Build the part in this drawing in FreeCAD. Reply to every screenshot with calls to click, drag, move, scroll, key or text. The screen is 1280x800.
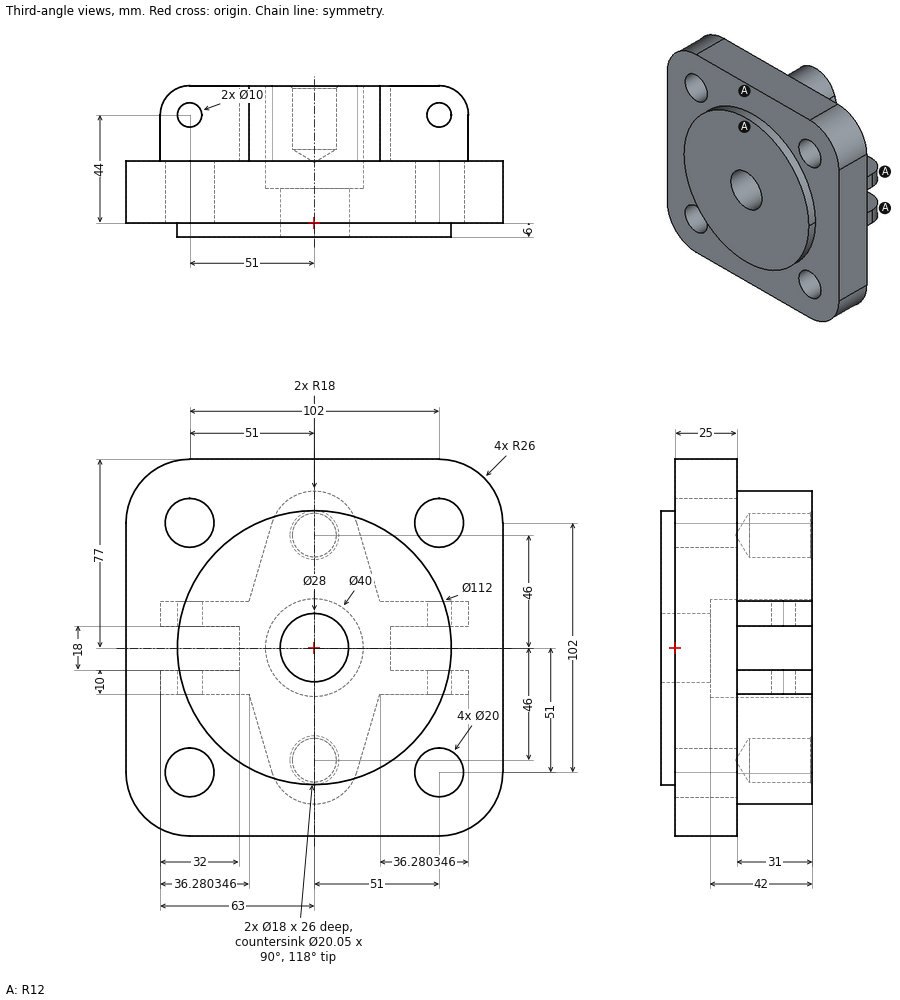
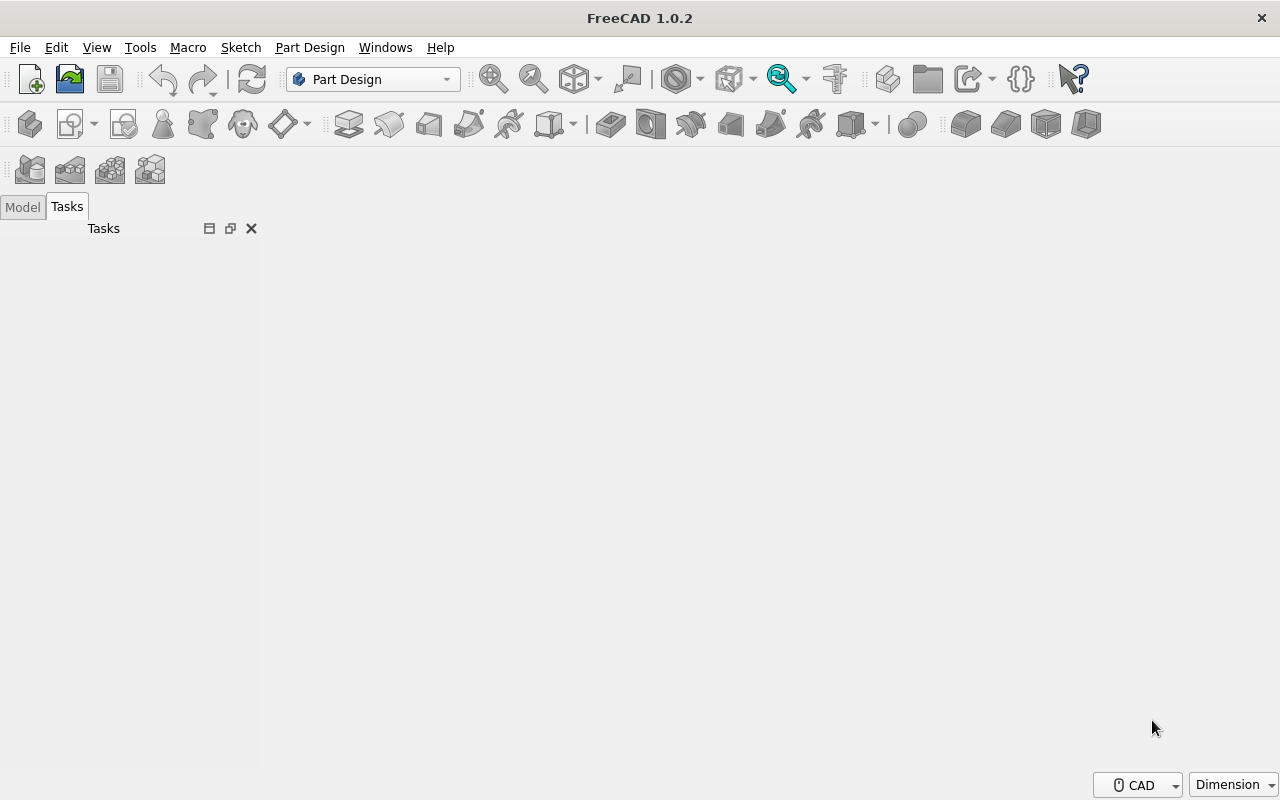
key(ctrl+n)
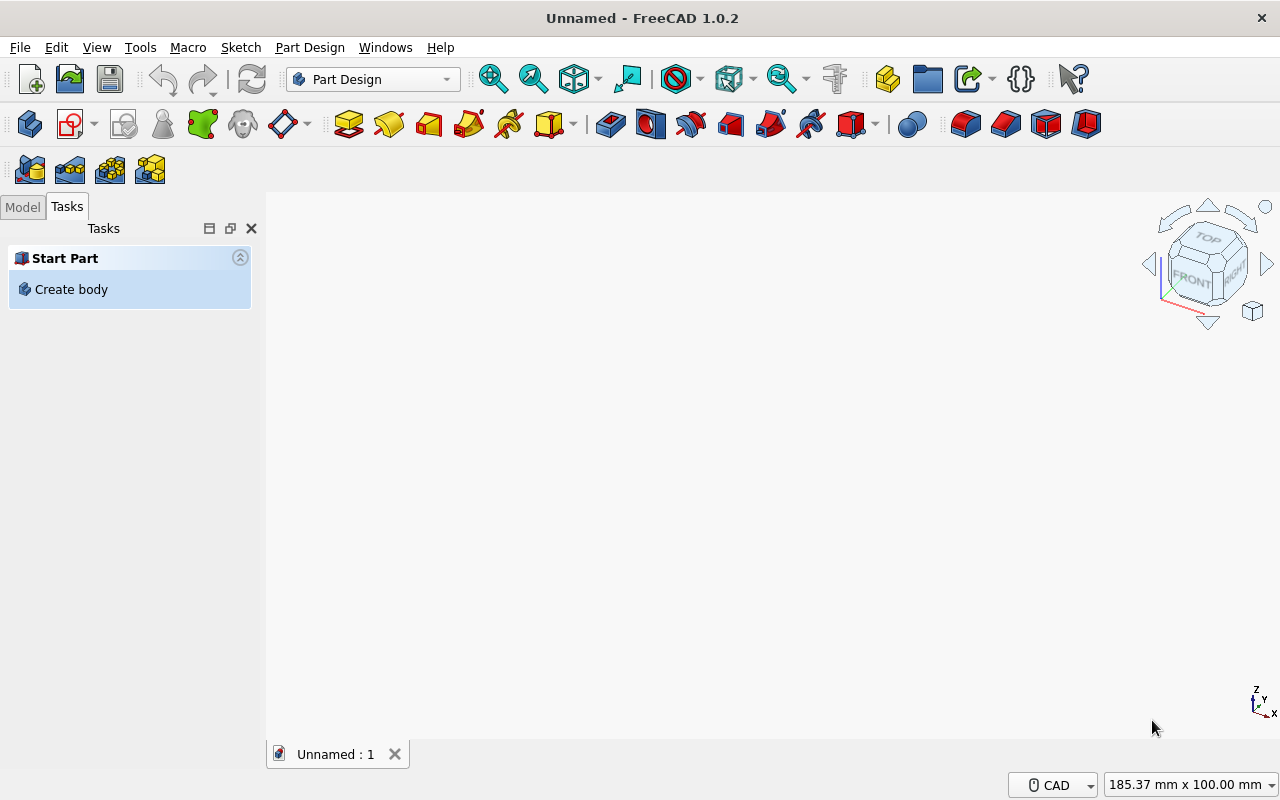
click(70, 124)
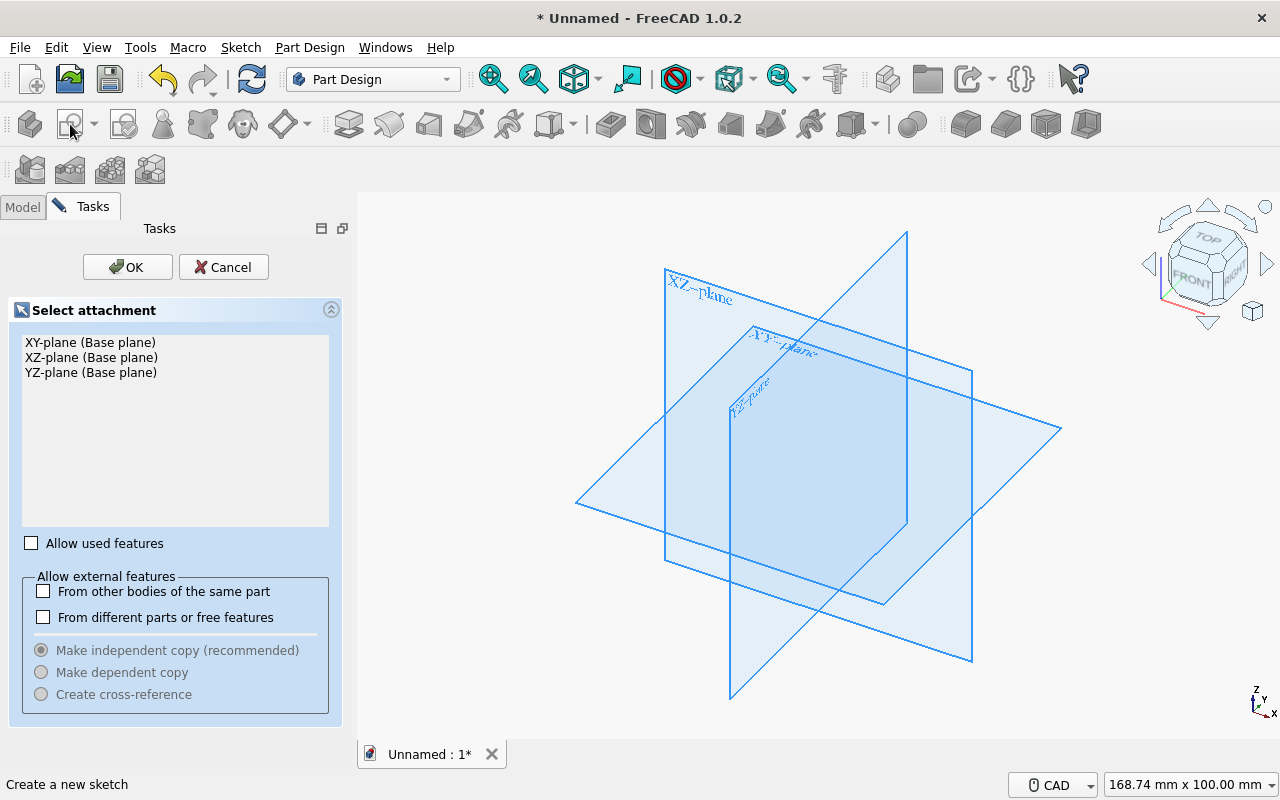
click(82, 358)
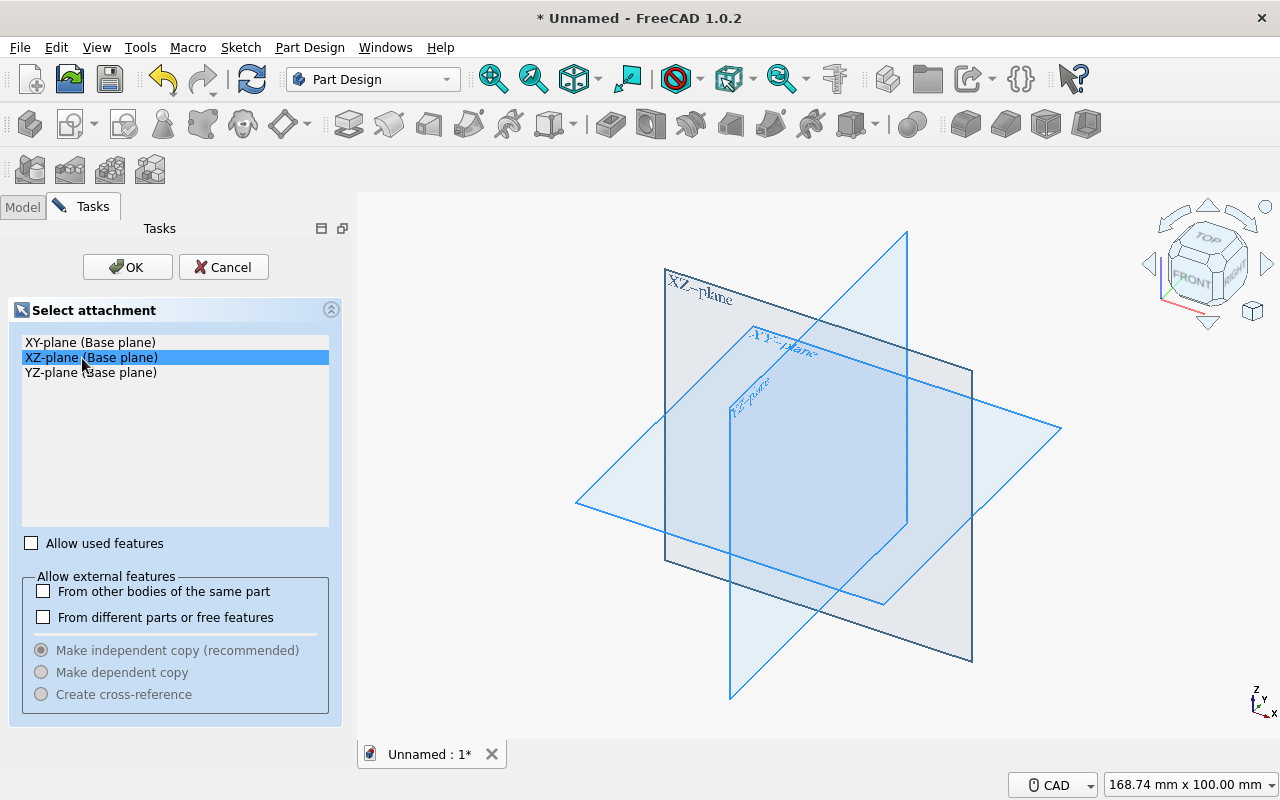
click(128, 267)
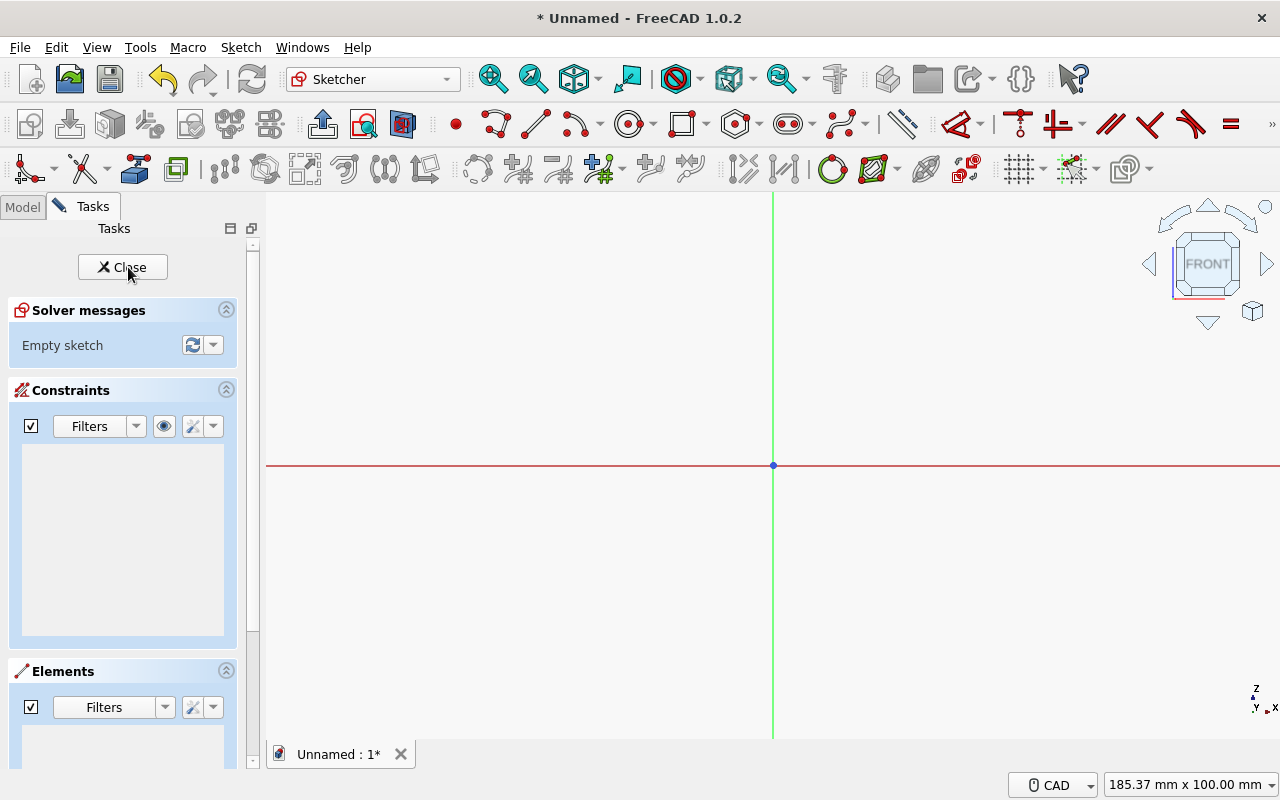
scroll(649, 466, down, 4)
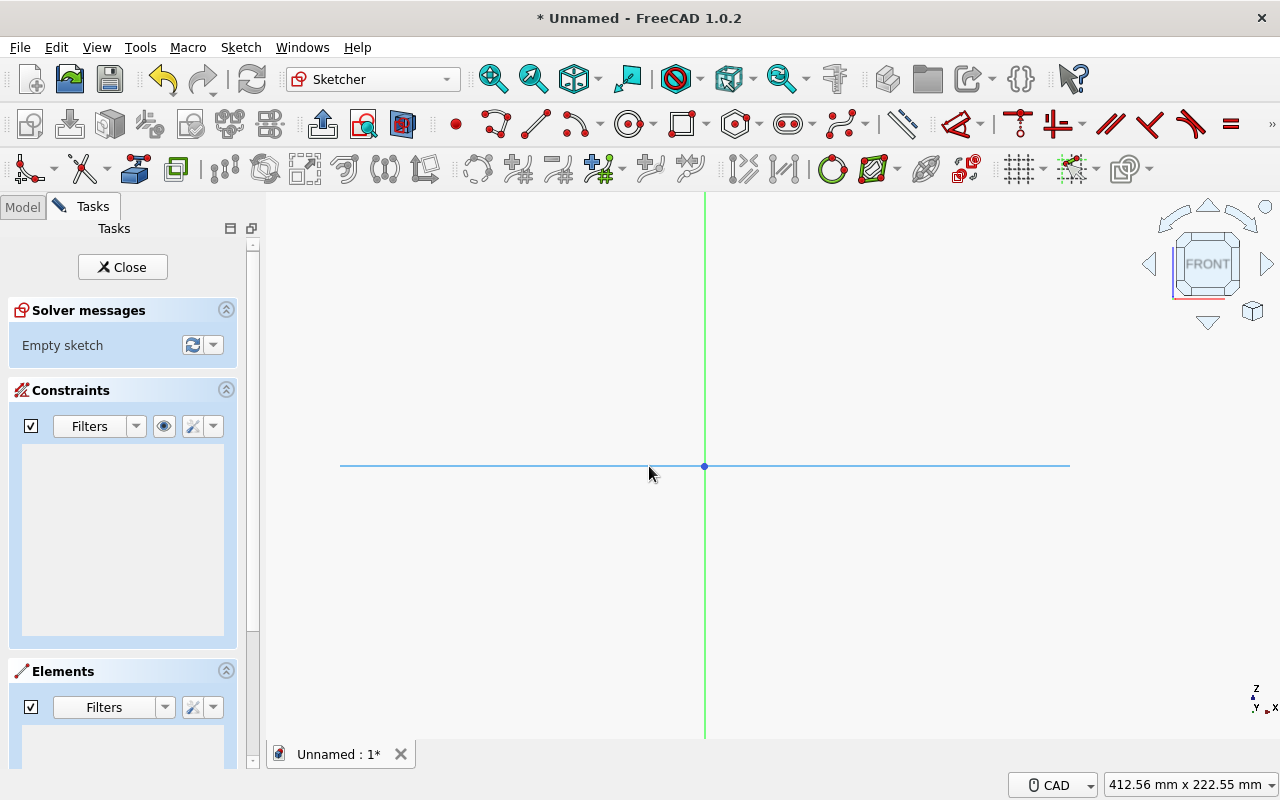
click(536, 124)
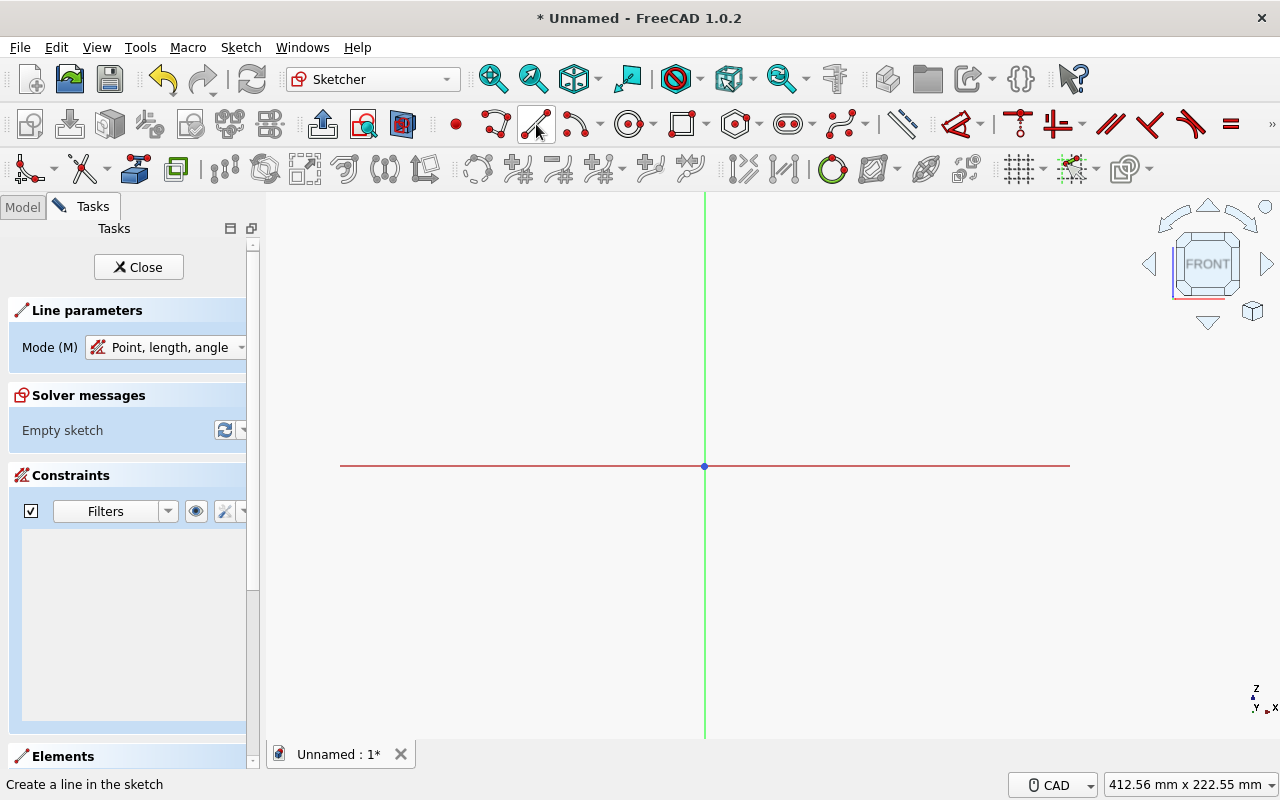
click(580, 277)
click(830, 277)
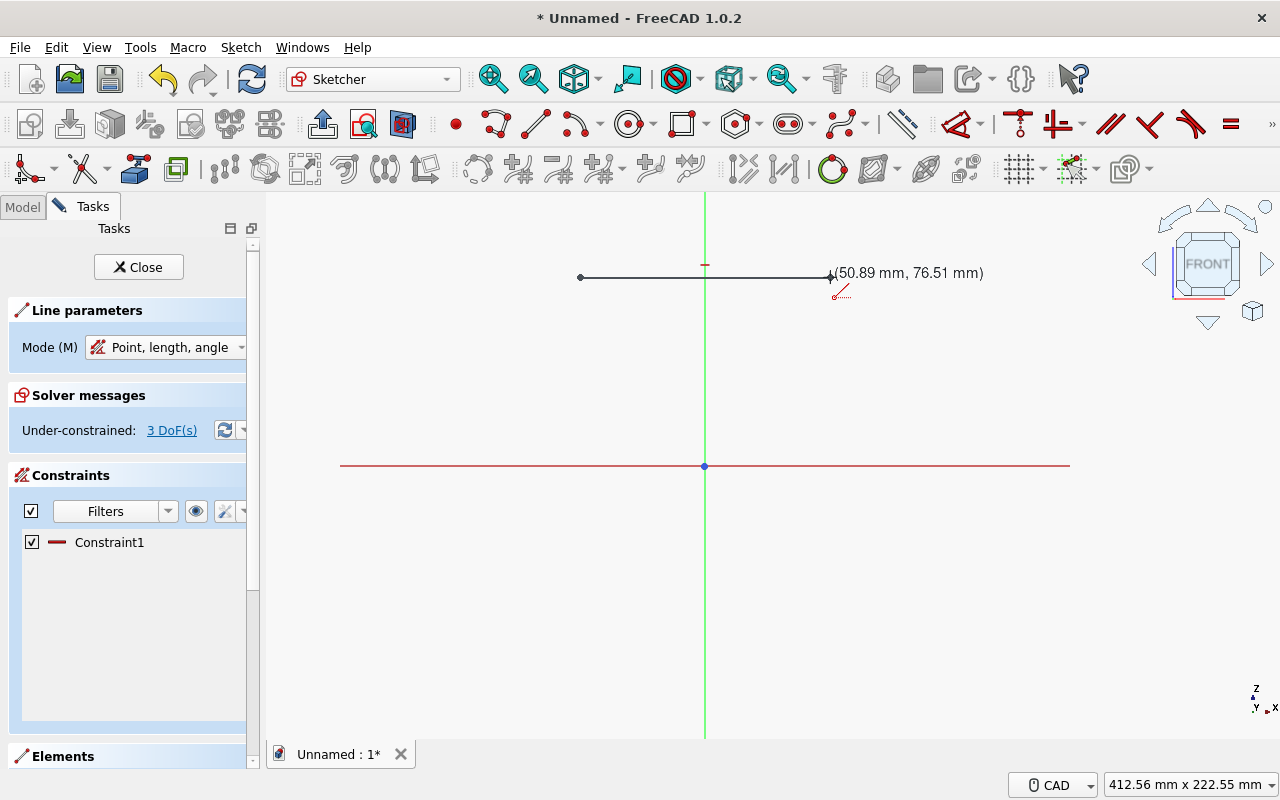
click(894, 341)
click(894, 591)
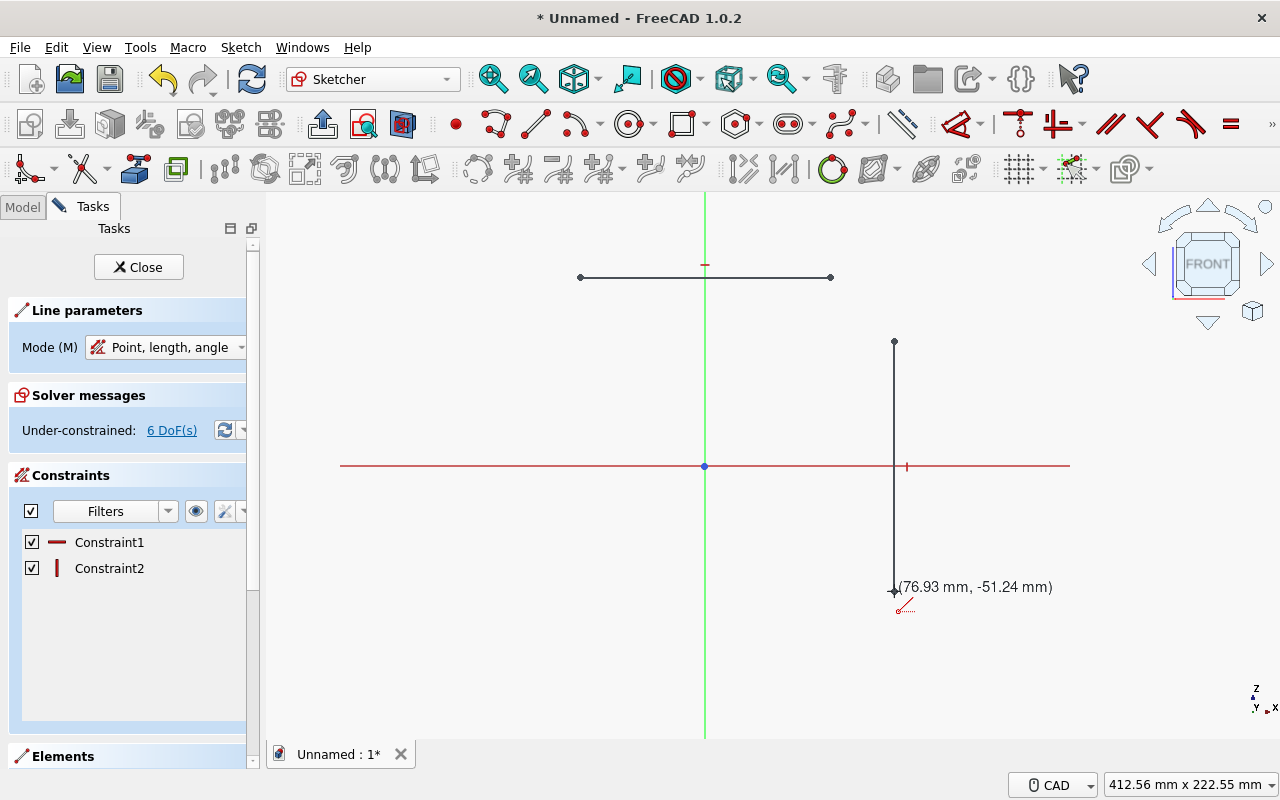
click(830, 655)
click(580, 655)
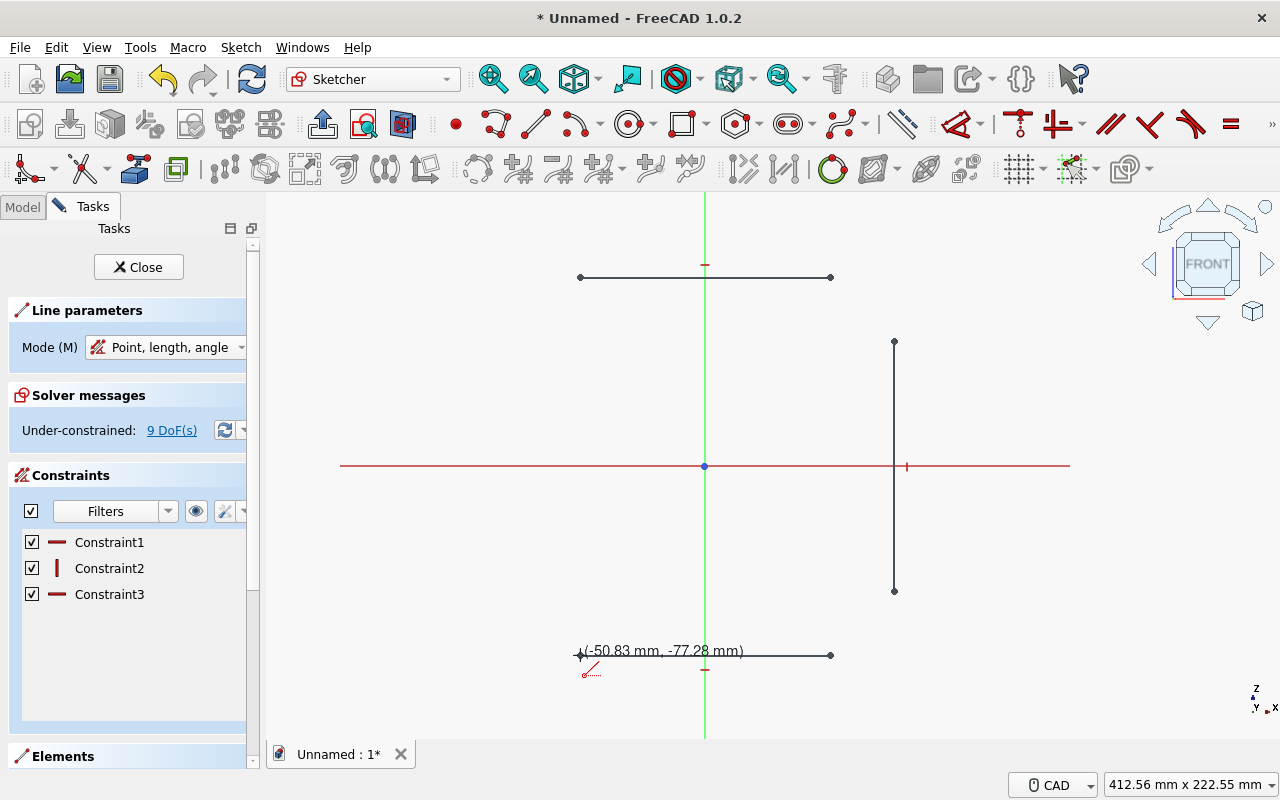
click(516, 591)
click(516, 341)